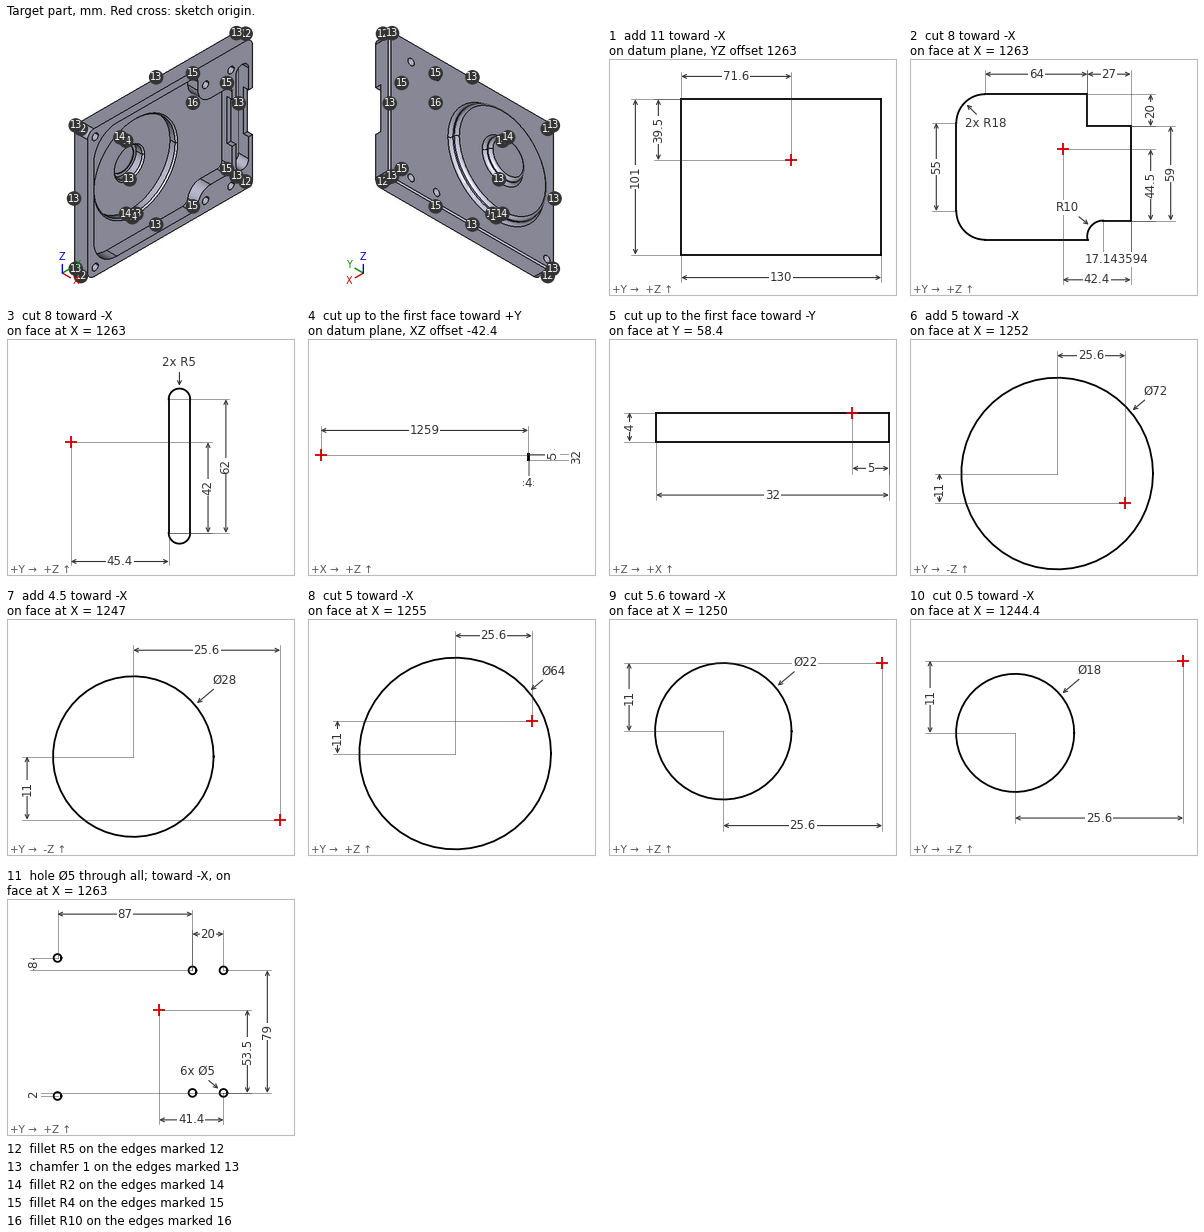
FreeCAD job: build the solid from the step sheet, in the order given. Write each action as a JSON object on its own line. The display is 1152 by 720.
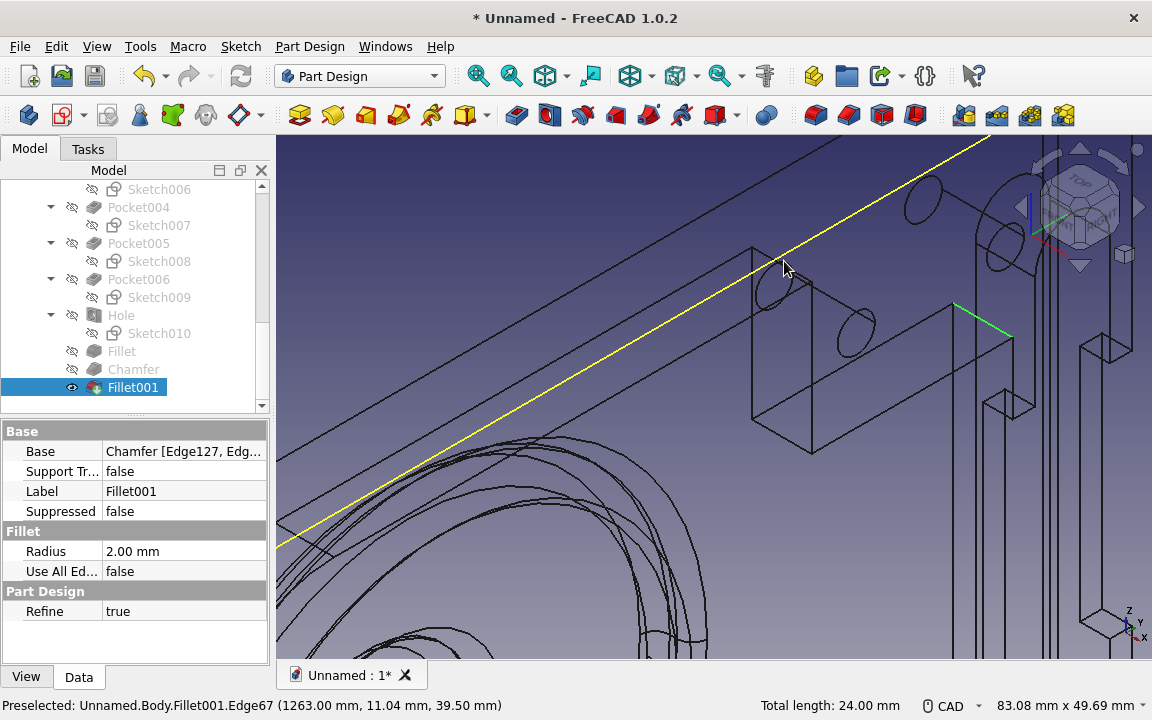
{"action": "left_click", "coordinate": [782, 263], "text": "ctrl"}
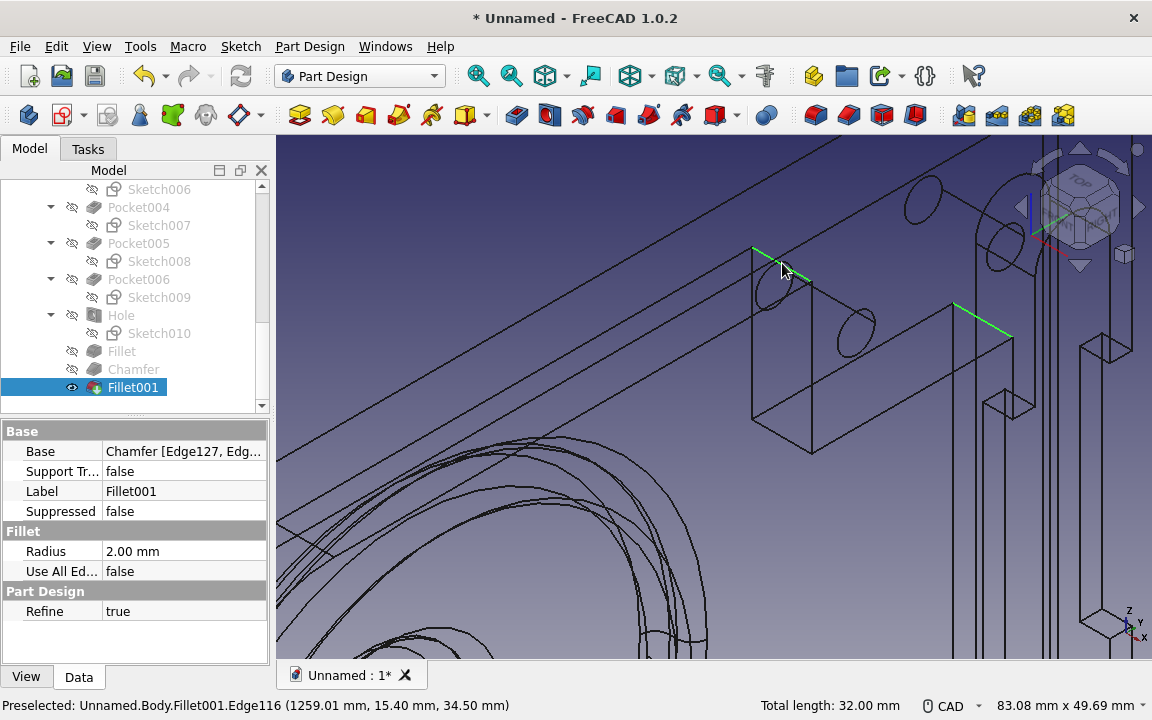
{"action": "key", "text": "v 1"}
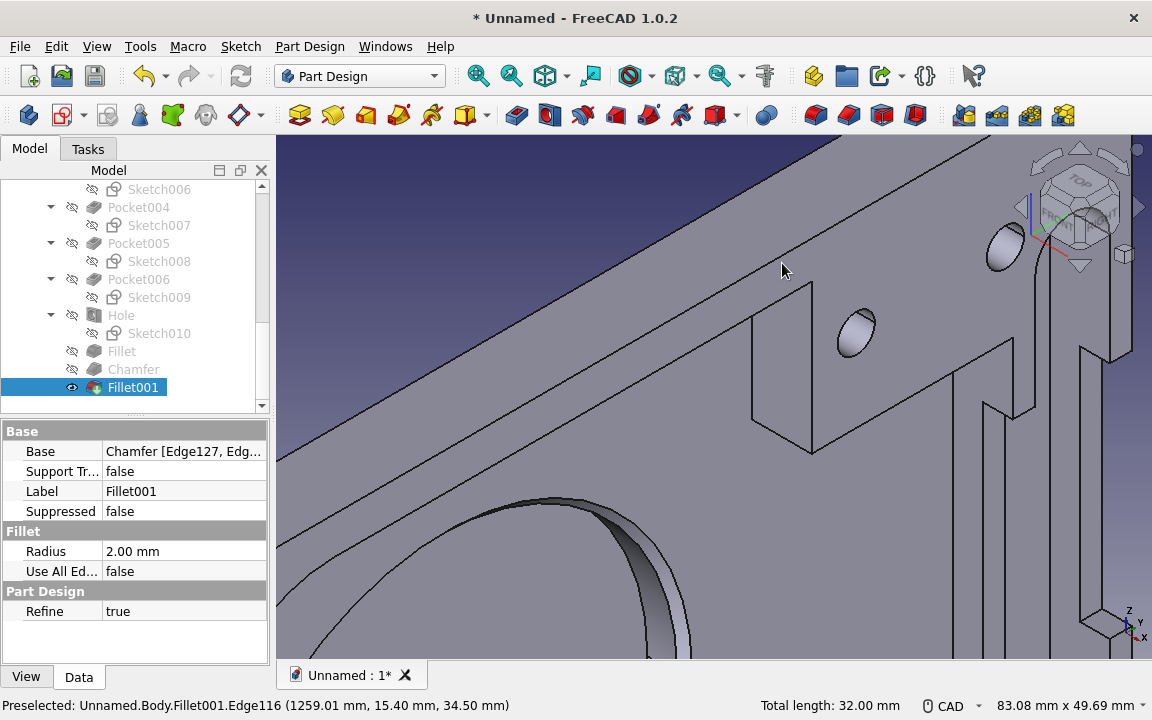
{"action": "left_click", "coordinate": [816, 116]}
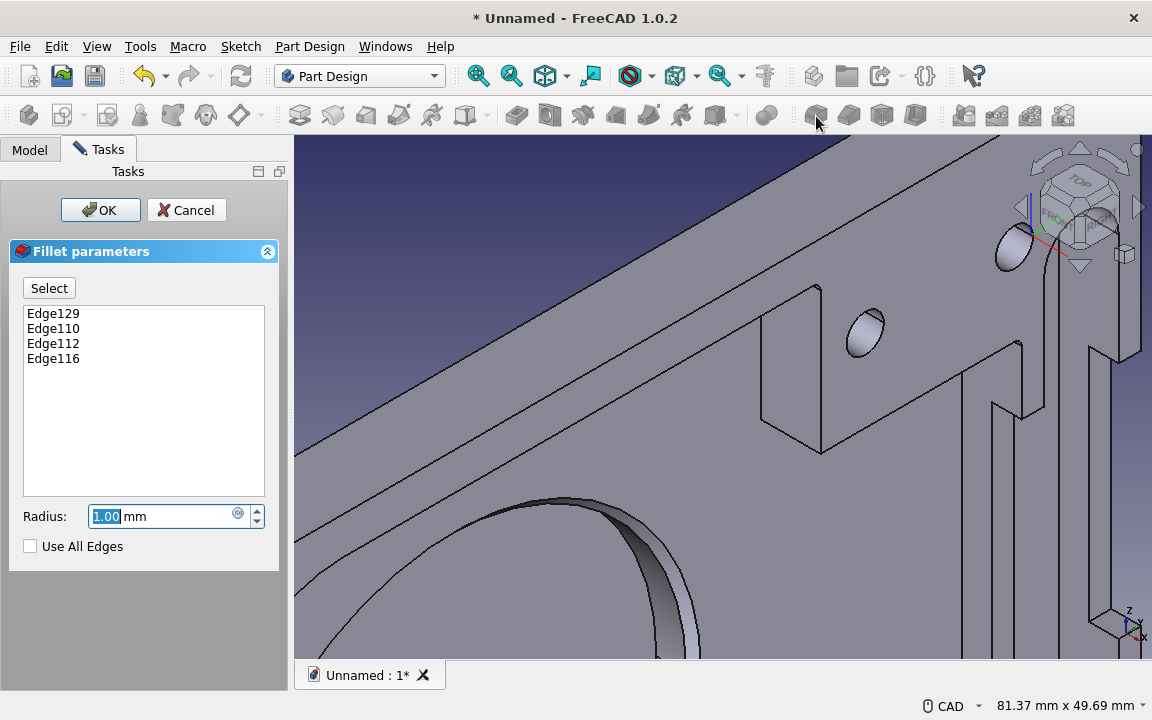
{"action": "type", "text": "4"}
{"action": "key", "text": "Tab"}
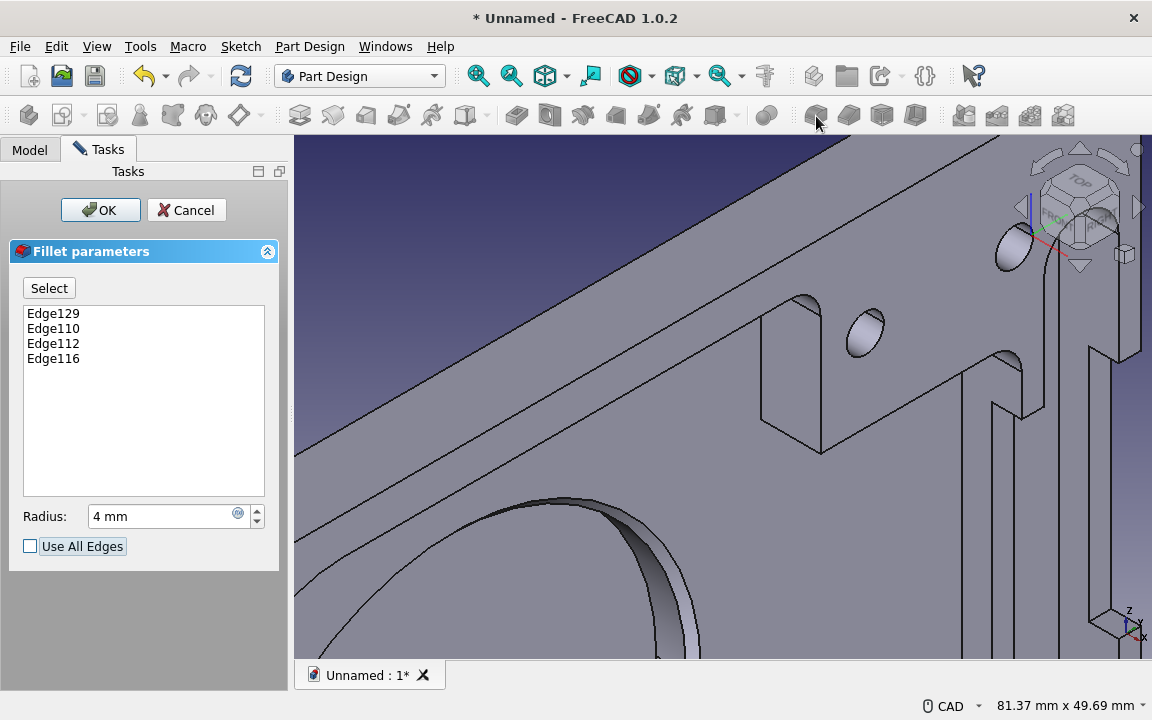
{"action": "left_click", "coordinate": [101, 210]}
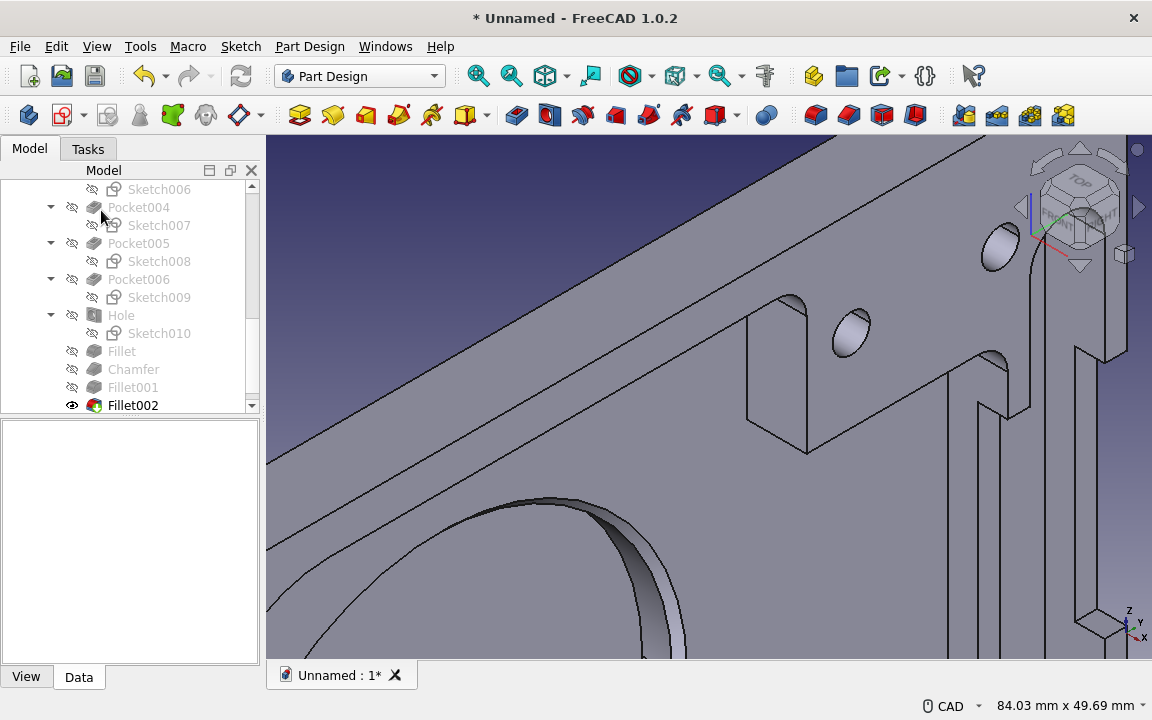
{"action": "left_click", "coordinate": [479, 76]}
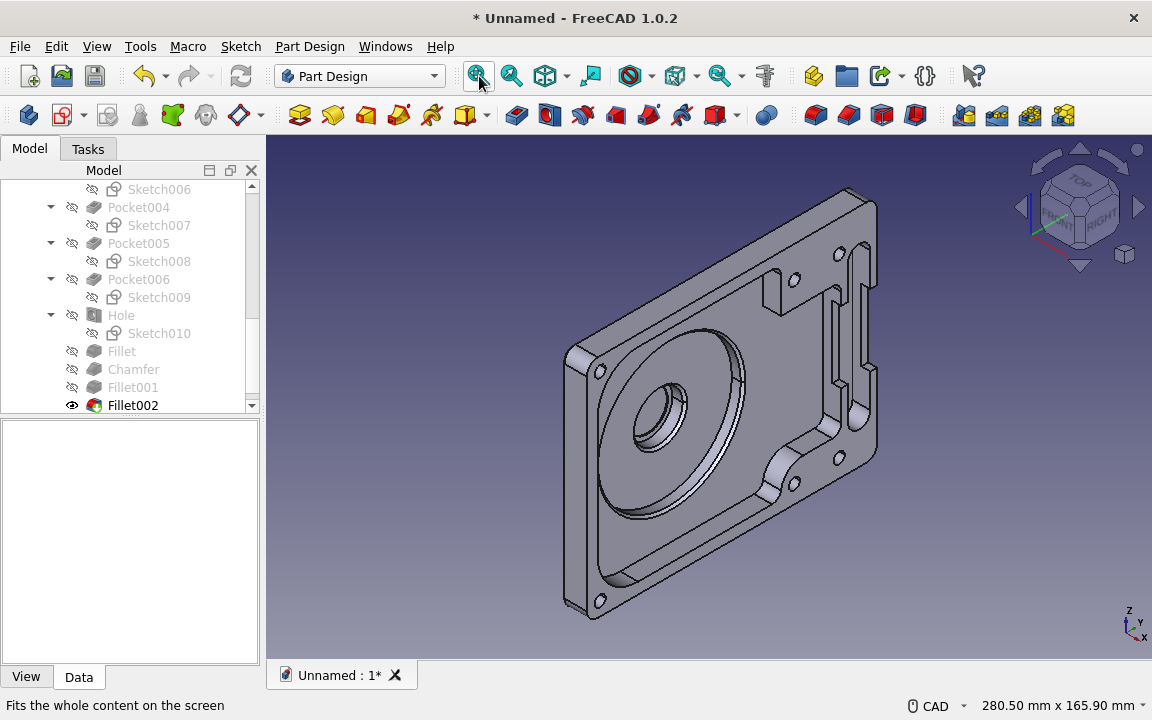
{"action": "key", "text": "2"}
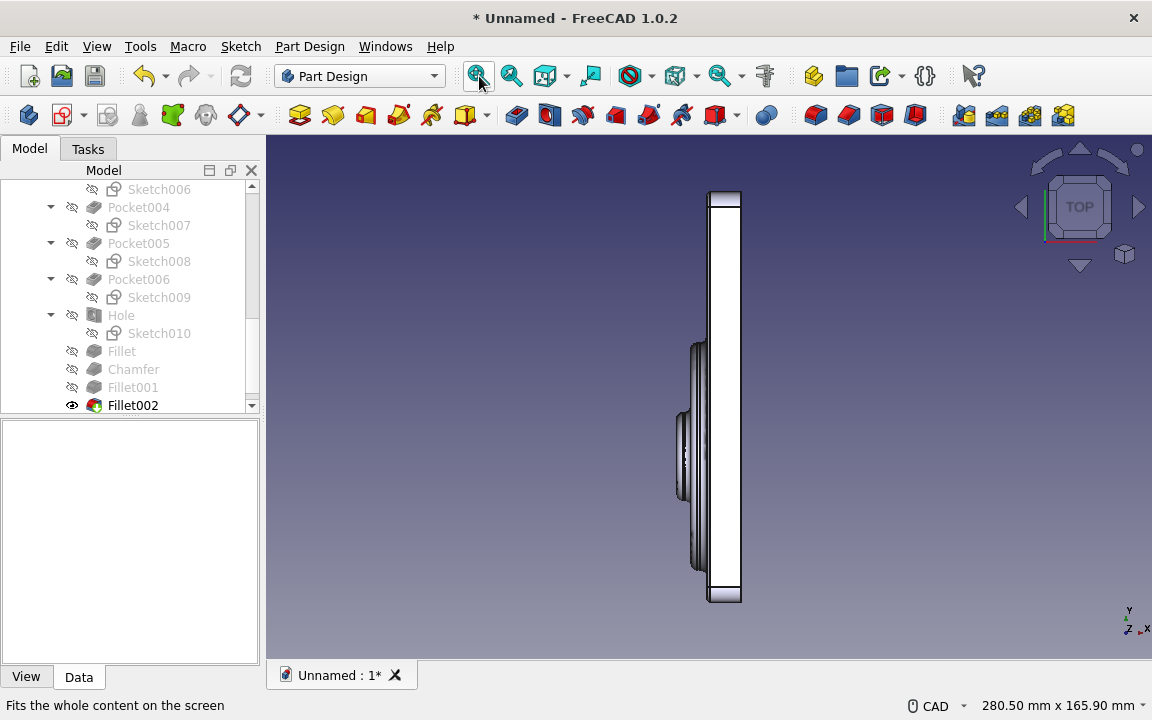
{"action": "key", "text": "0"}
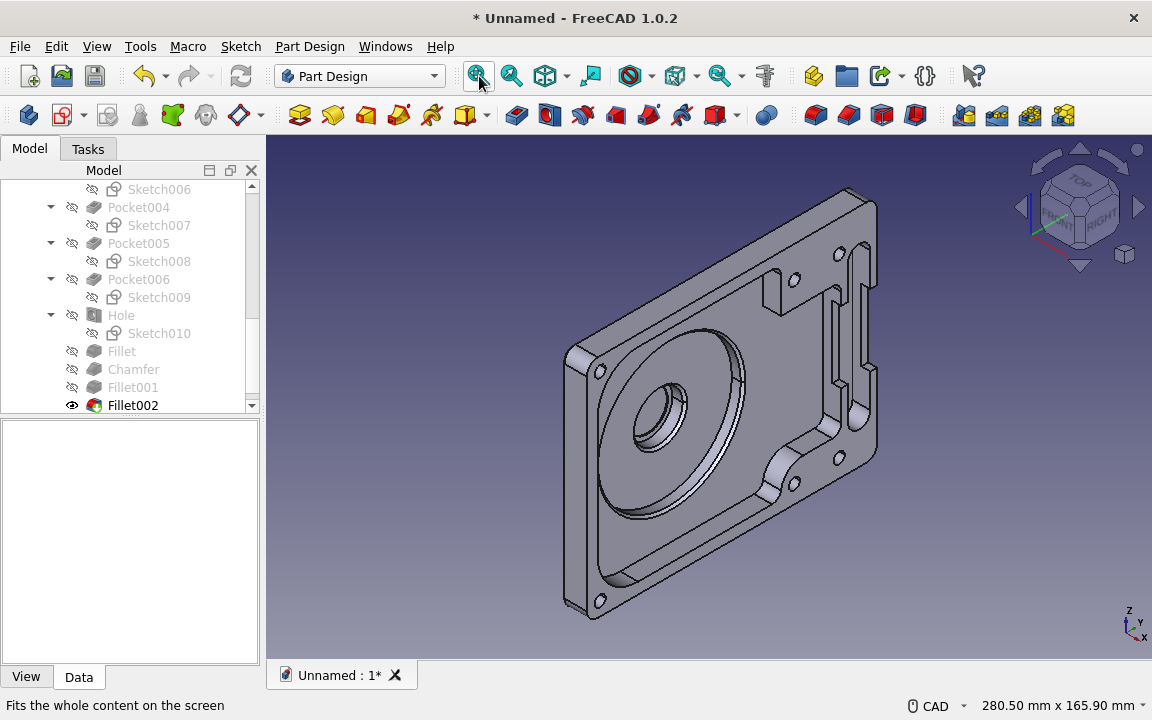
{"action": "key", "text": "1"}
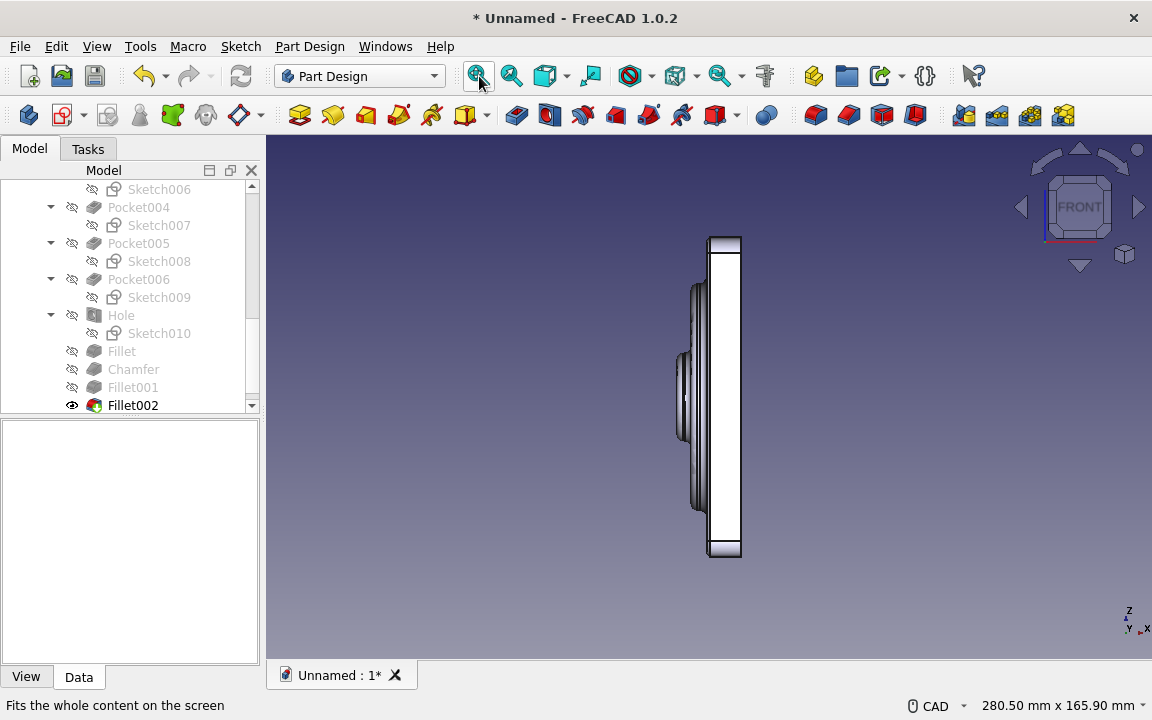
{"action": "key", "text": "3"}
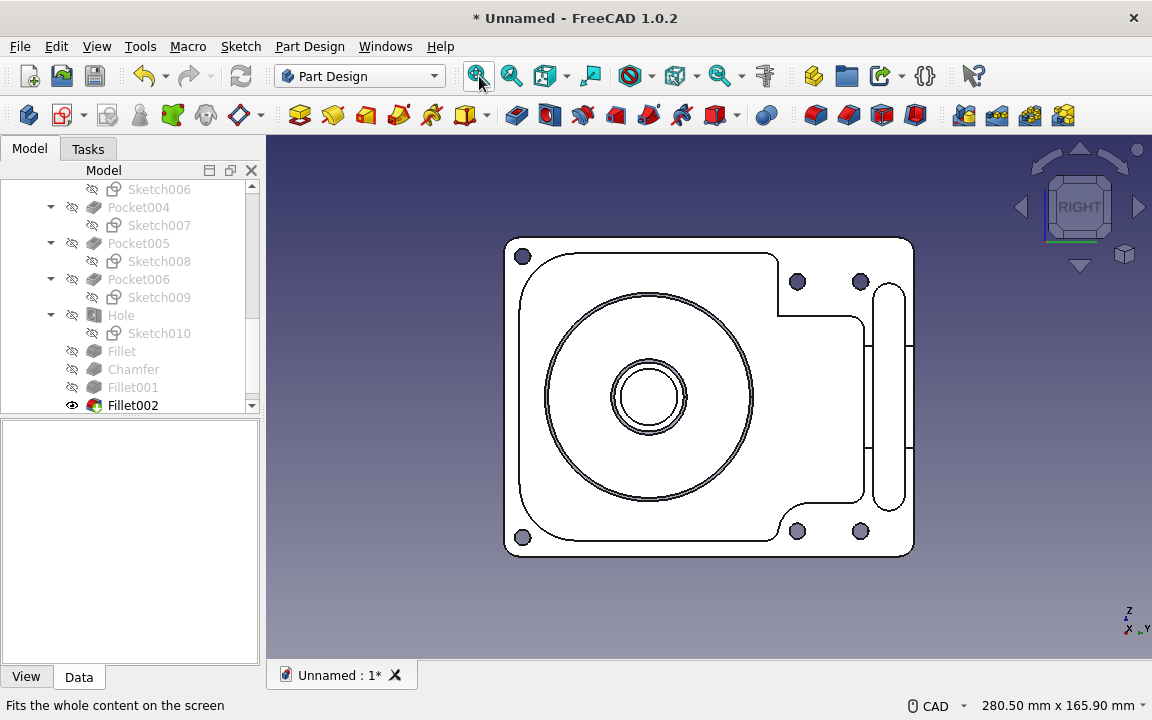
{"action": "key", "text": "5"}